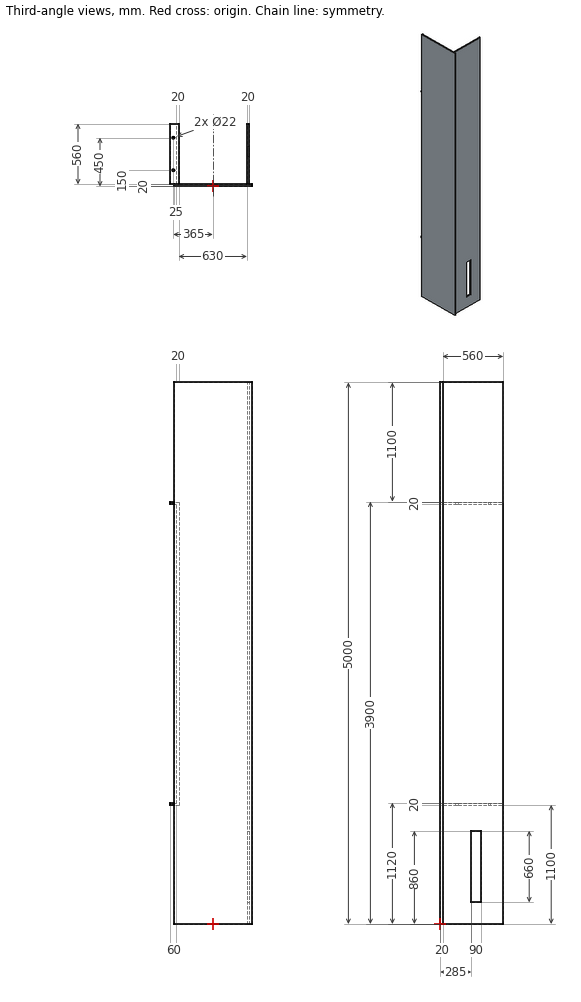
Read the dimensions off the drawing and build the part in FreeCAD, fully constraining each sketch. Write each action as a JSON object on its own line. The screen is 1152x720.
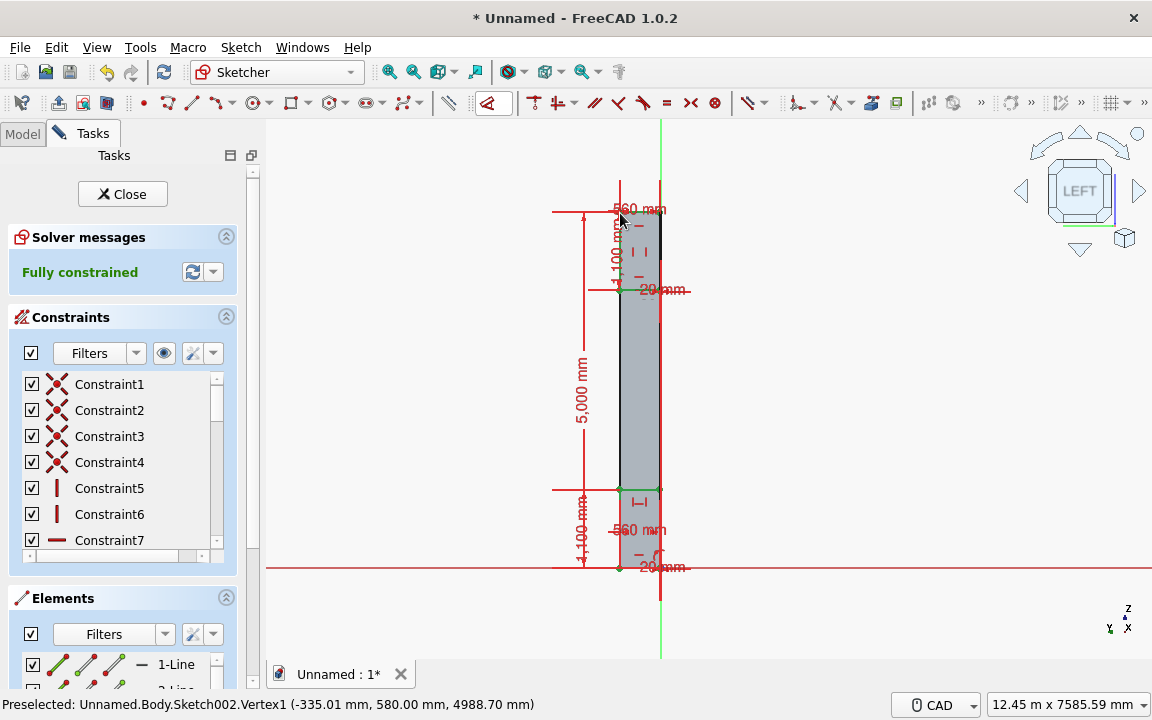
{"action": "left_click", "coordinate": [123, 194]}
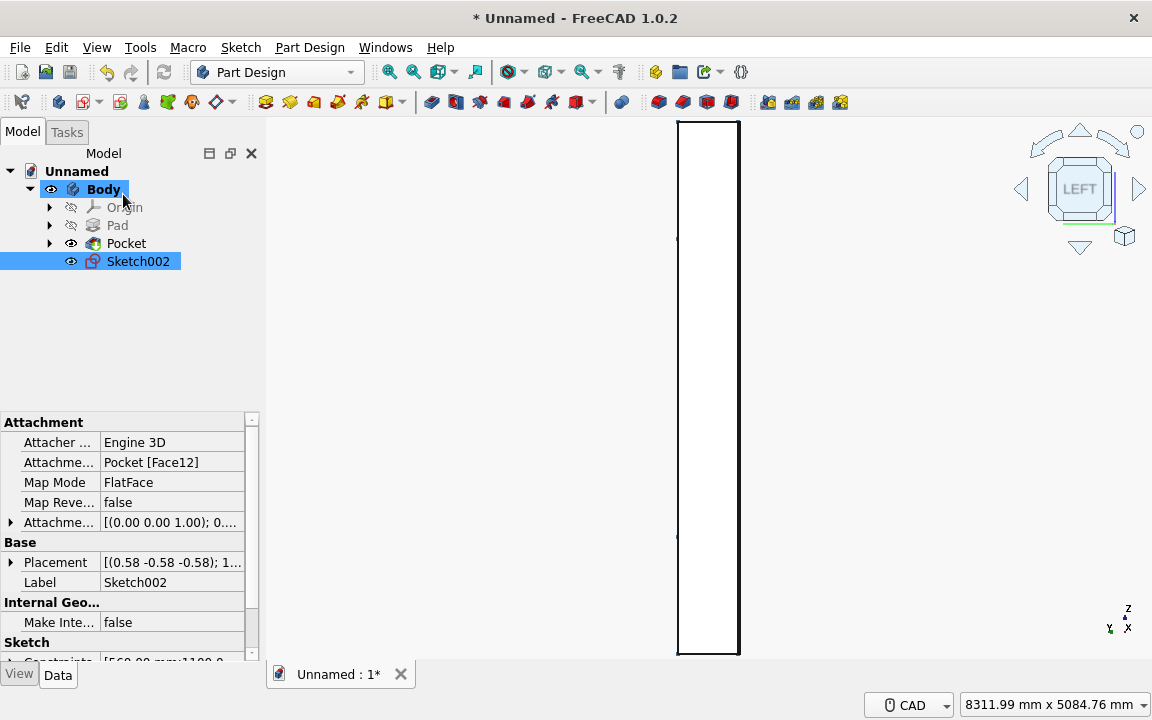
{"action": "left_click", "coordinate": [432, 102]}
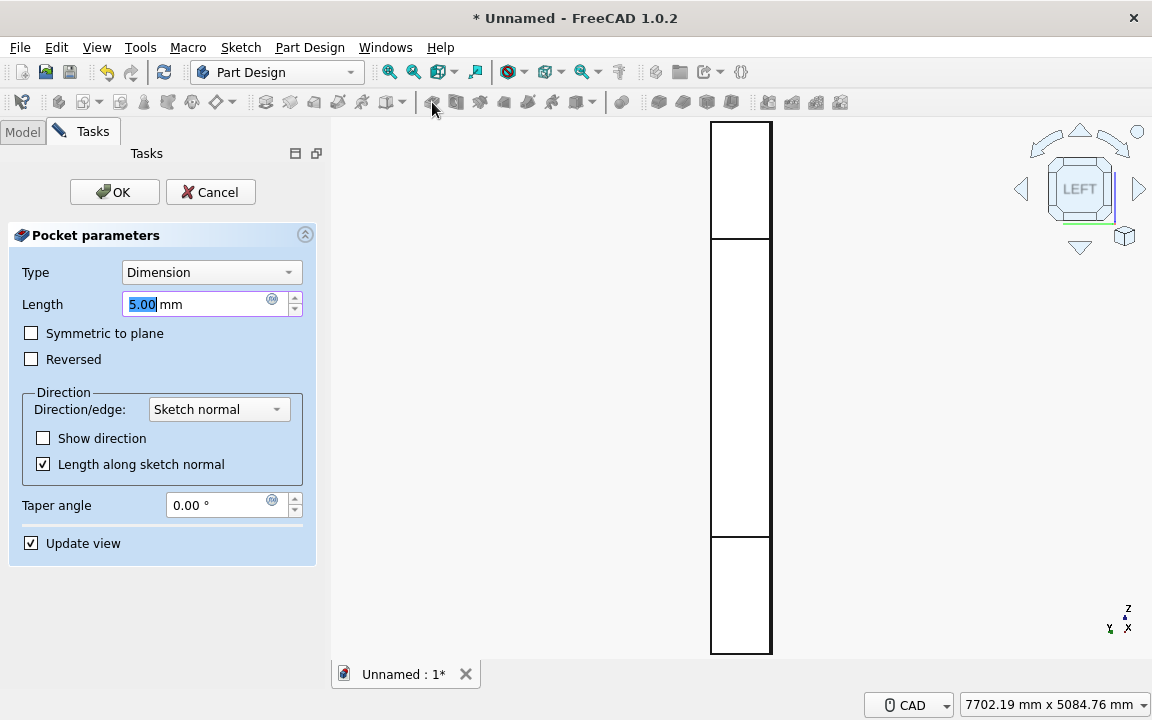
{"action": "type", "text": "20"}
{"action": "key", "text": "Tab"}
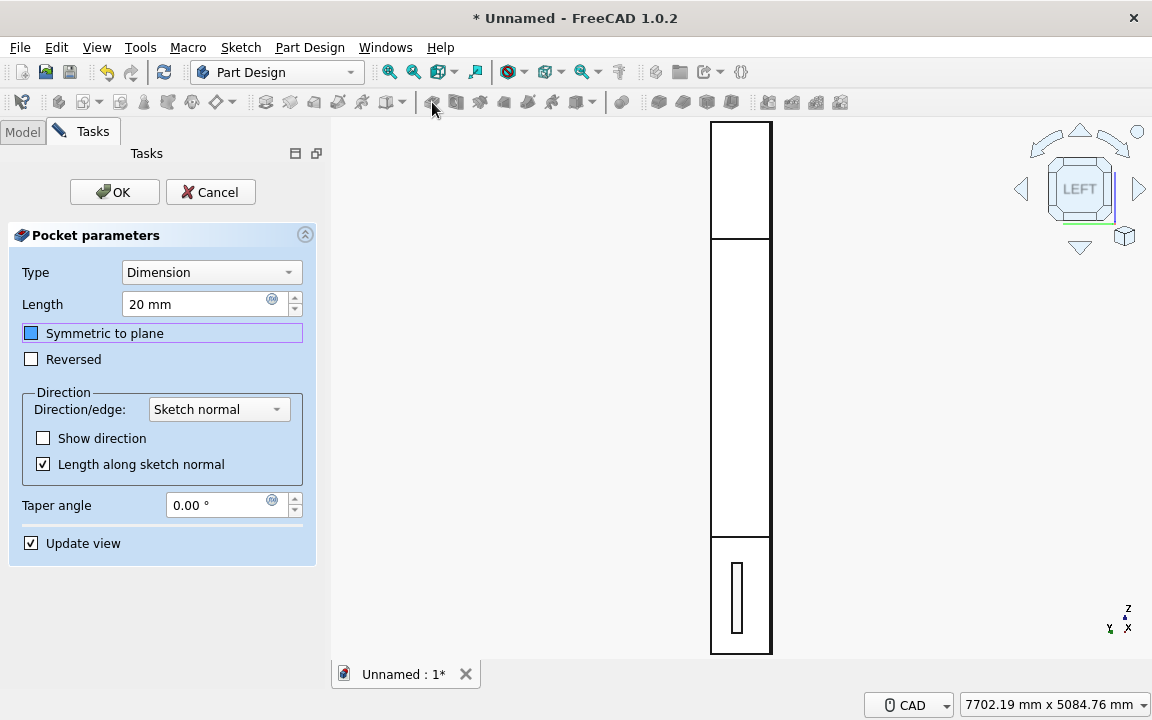
{"action": "left_click", "coordinate": [115, 192]}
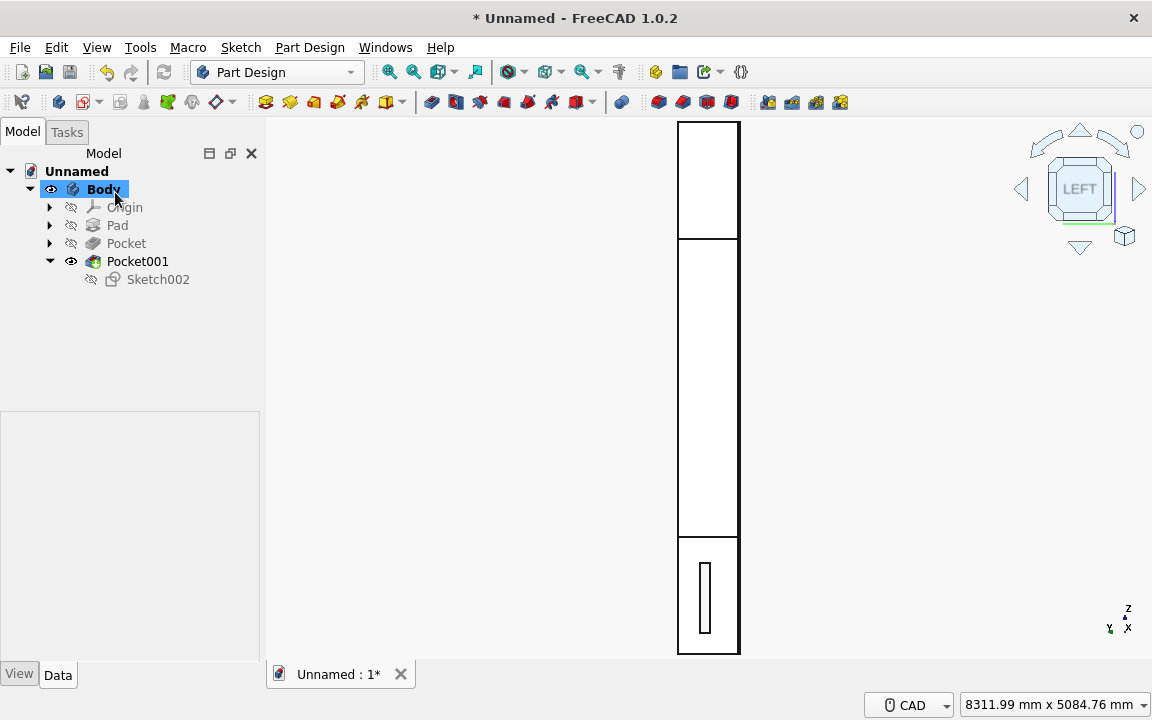
{"action": "left_click", "coordinate": [708, 302]}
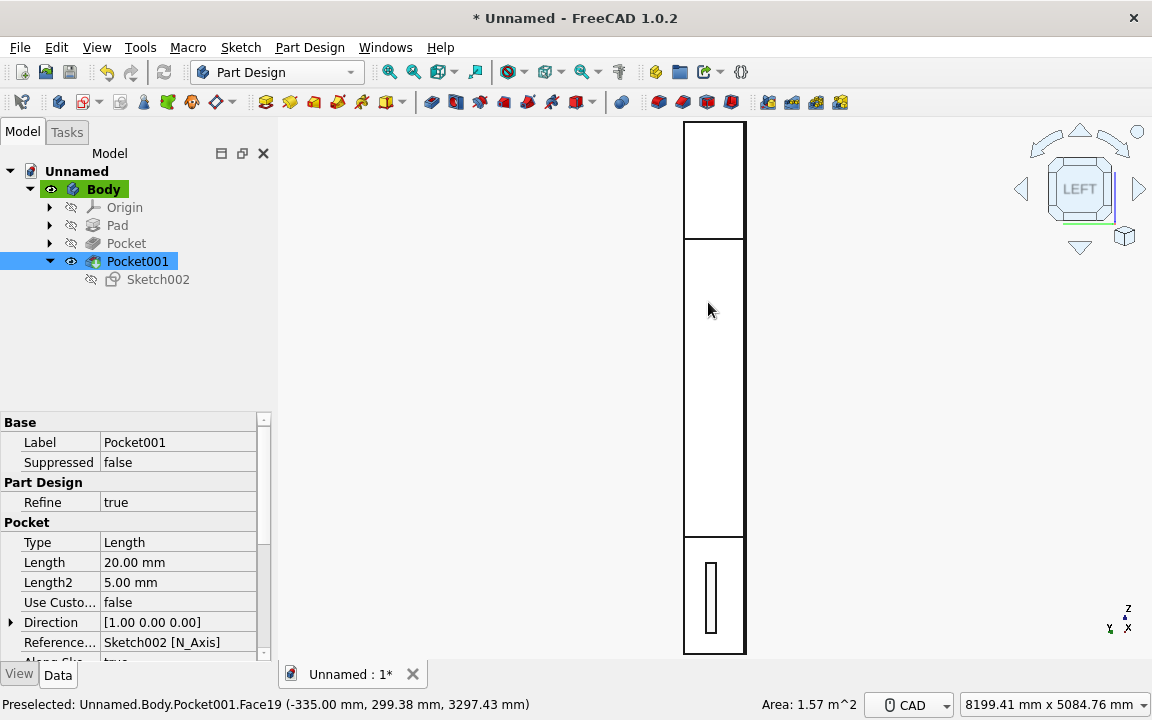
{"action": "left_click", "coordinate": [84, 102]}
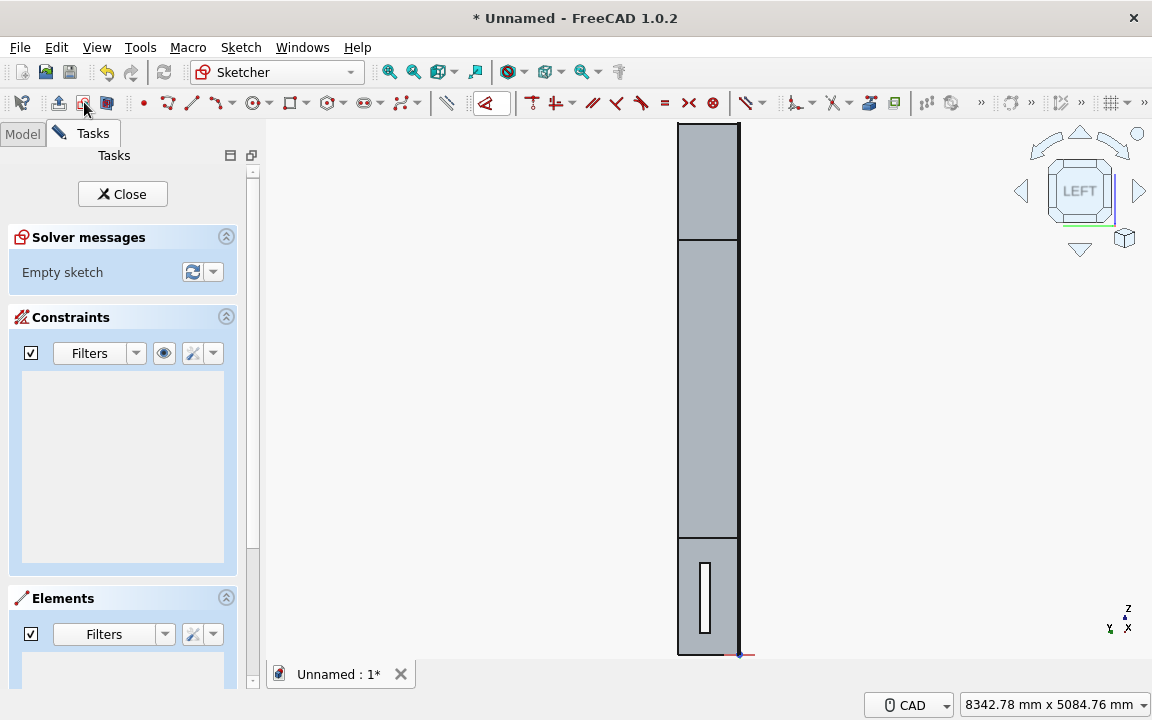
{"action": "left_click", "coordinate": [108, 104]}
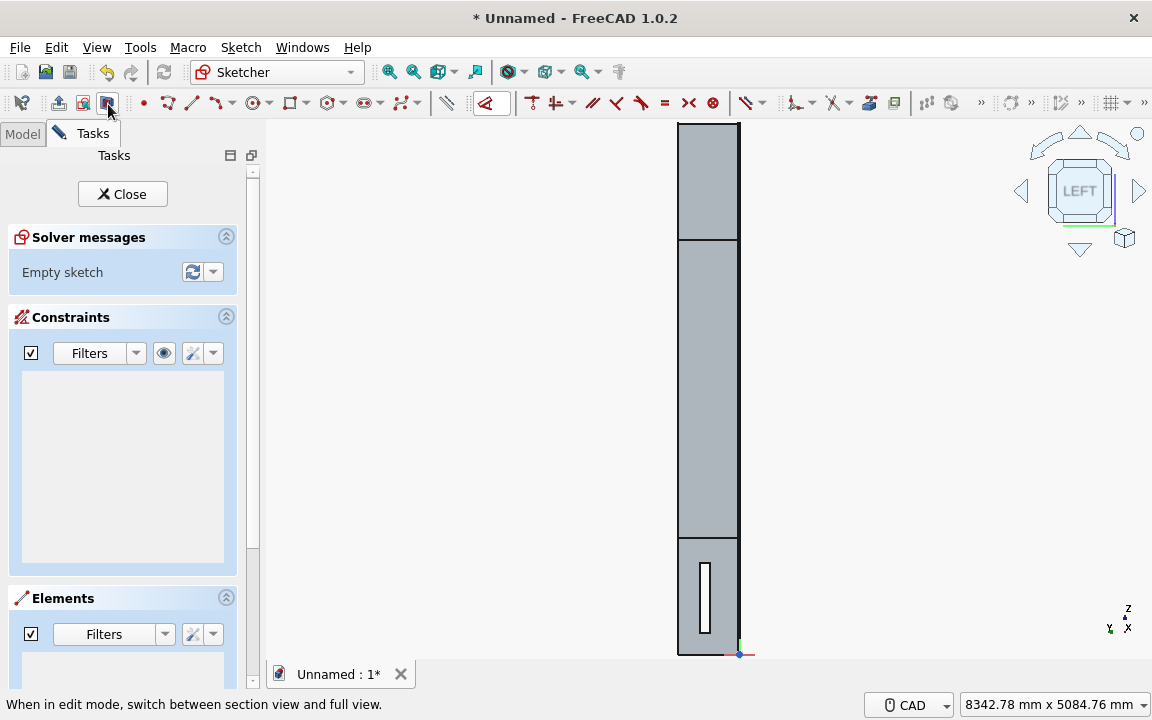
{"action": "scroll", "coordinate": [331, 147], "scroll_direction": "down", "scroll_amount": 1}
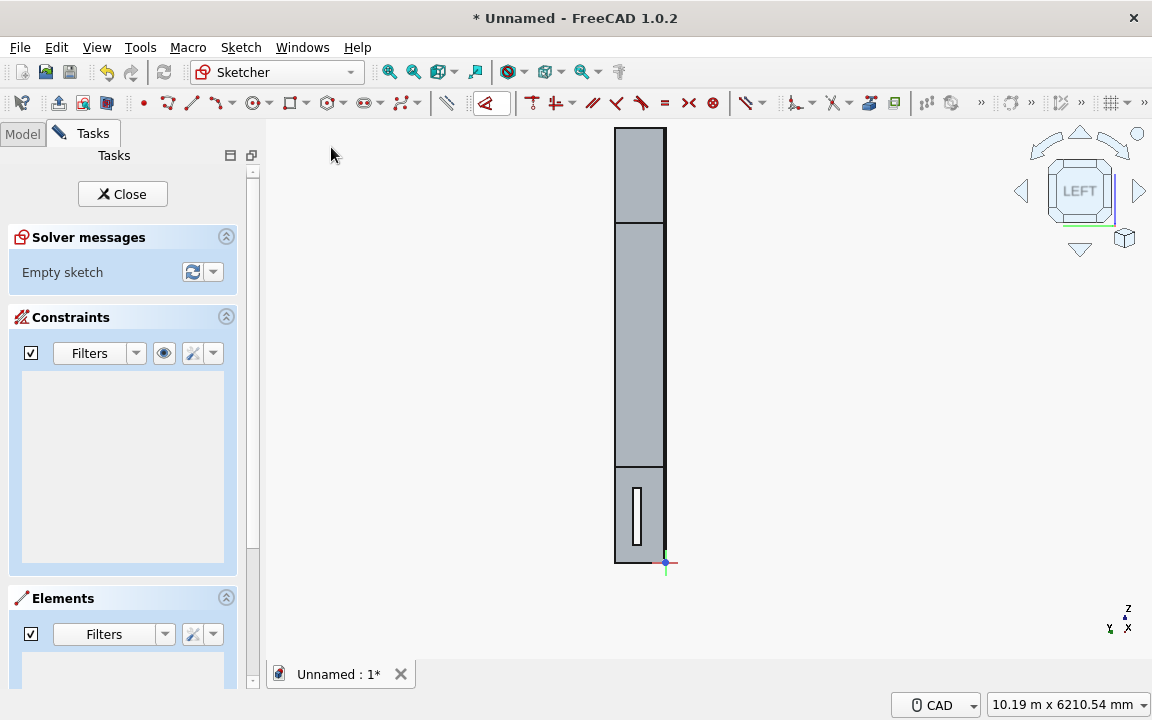
{"action": "left_click", "coordinate": [290, 104]}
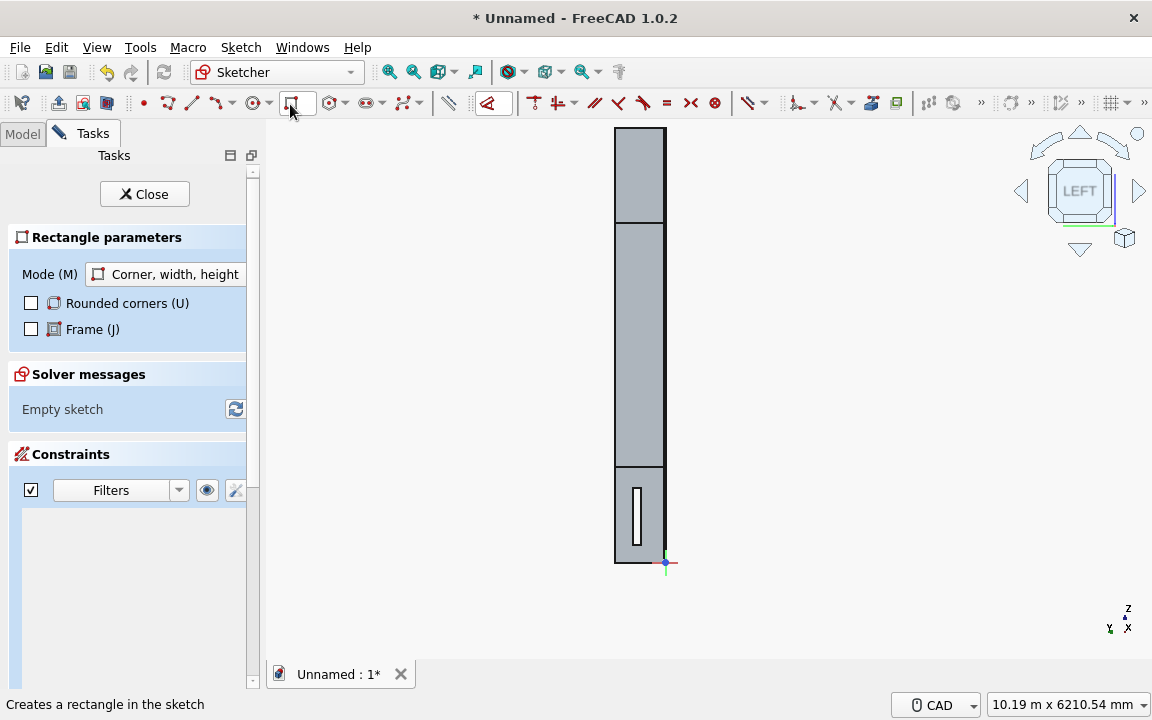
{"action": "scroll", "coordinate": [615, 465], "scroll_direction": "up", "scroll_amount": 12}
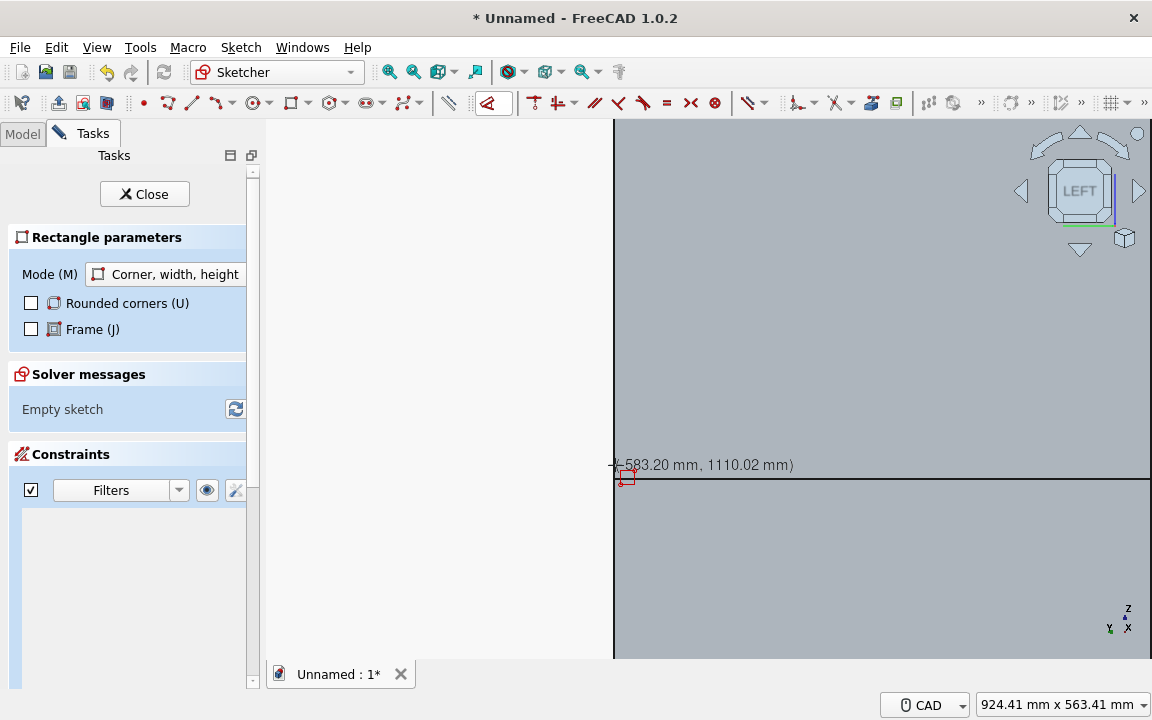
{"action": "scroll", "coordinate": [615, 461], "scroll_direction": "down", "scroll_amount": 12}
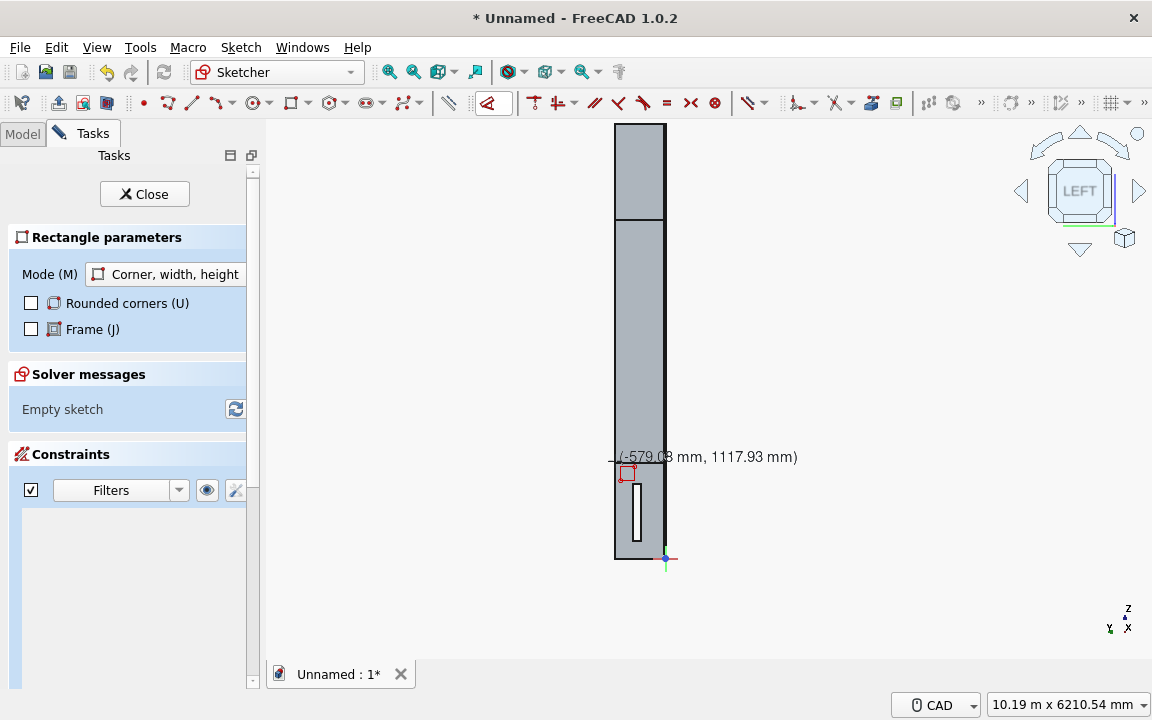
{"action": "left_click", "coordinate": [615, 461]}